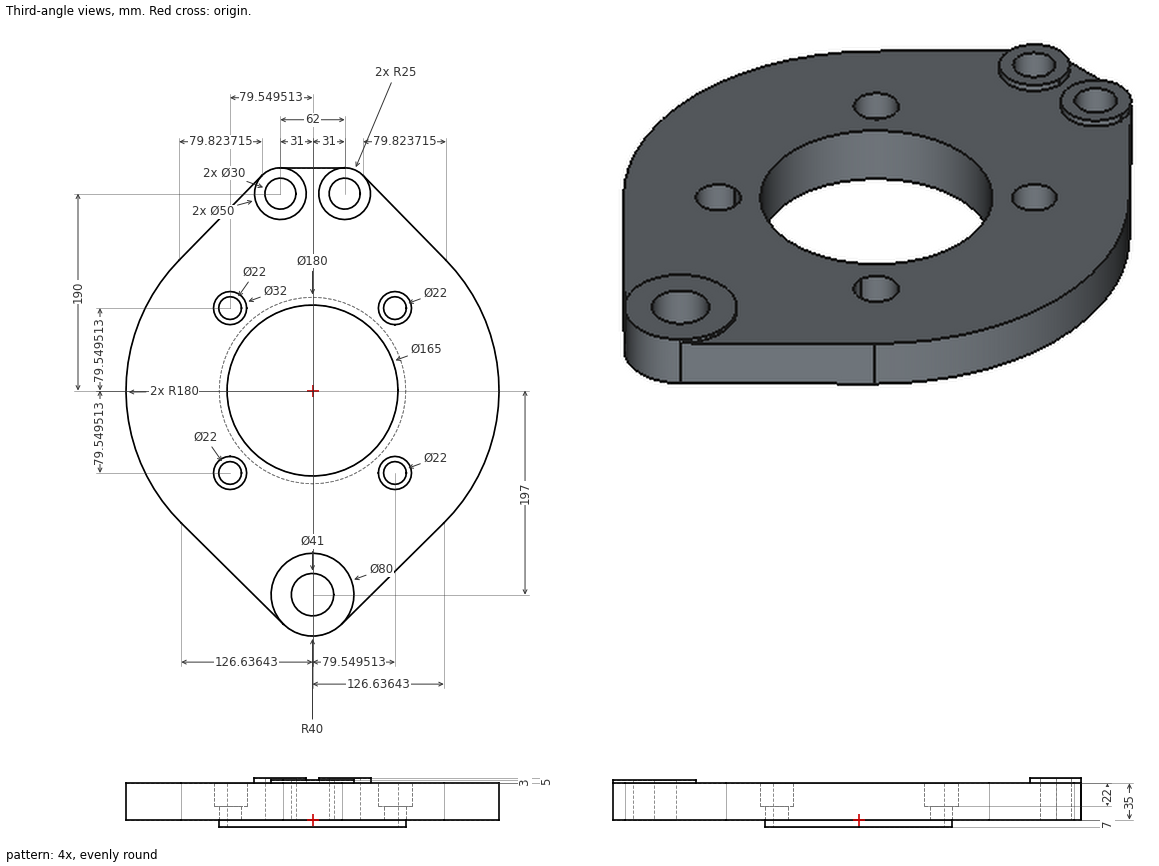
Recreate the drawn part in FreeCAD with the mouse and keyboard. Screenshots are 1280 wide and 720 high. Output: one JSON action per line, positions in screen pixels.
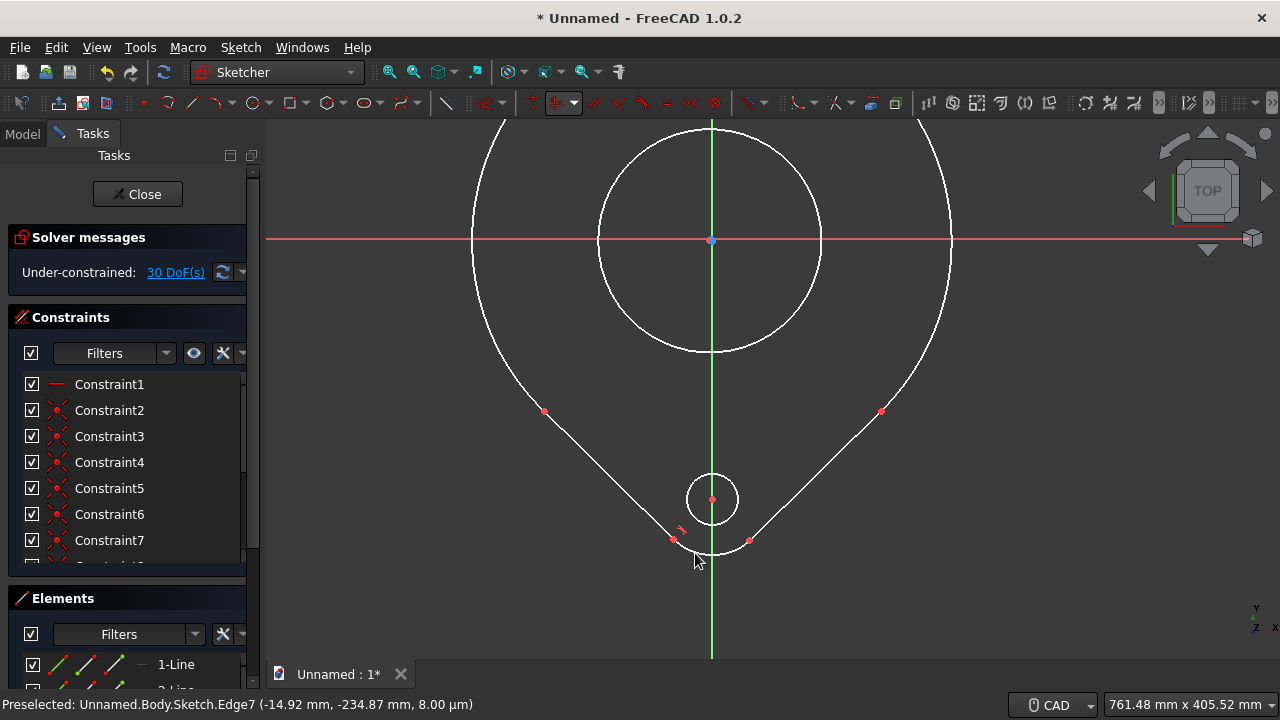
{"action": "left_click", "coordinate": [789, 502]}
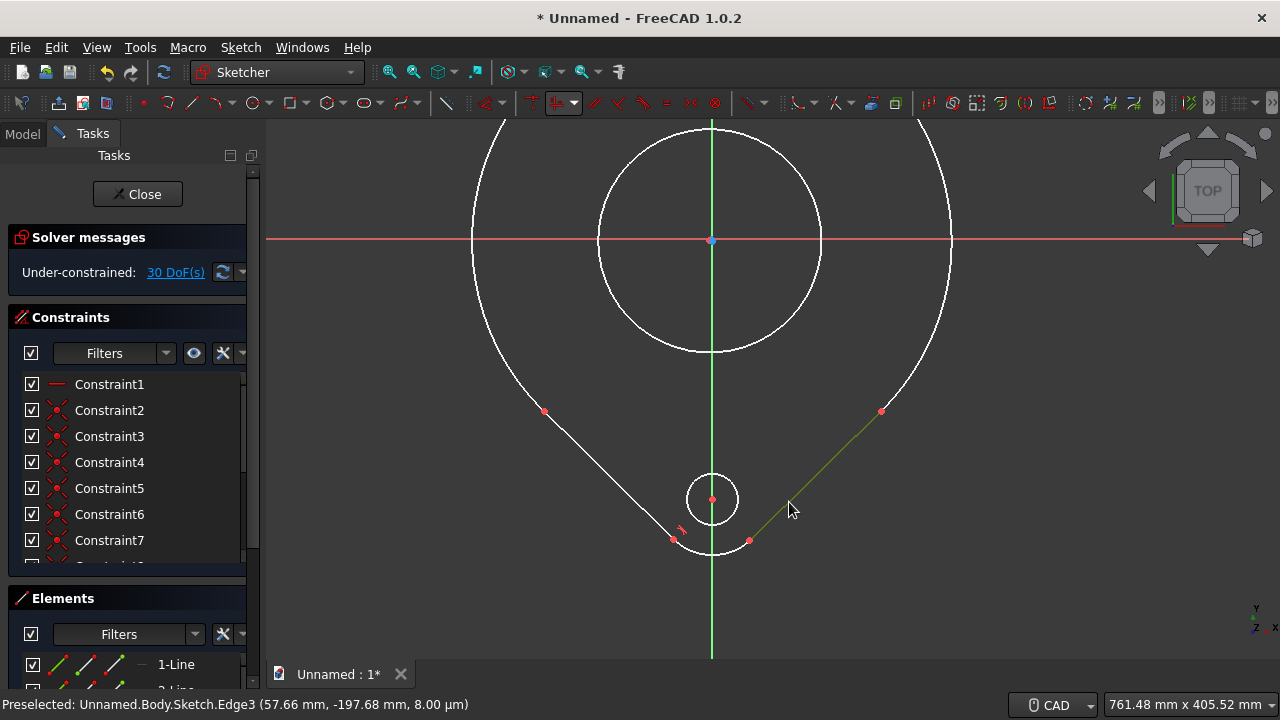
{"action": "left_click", "coordinate": [695, 552]}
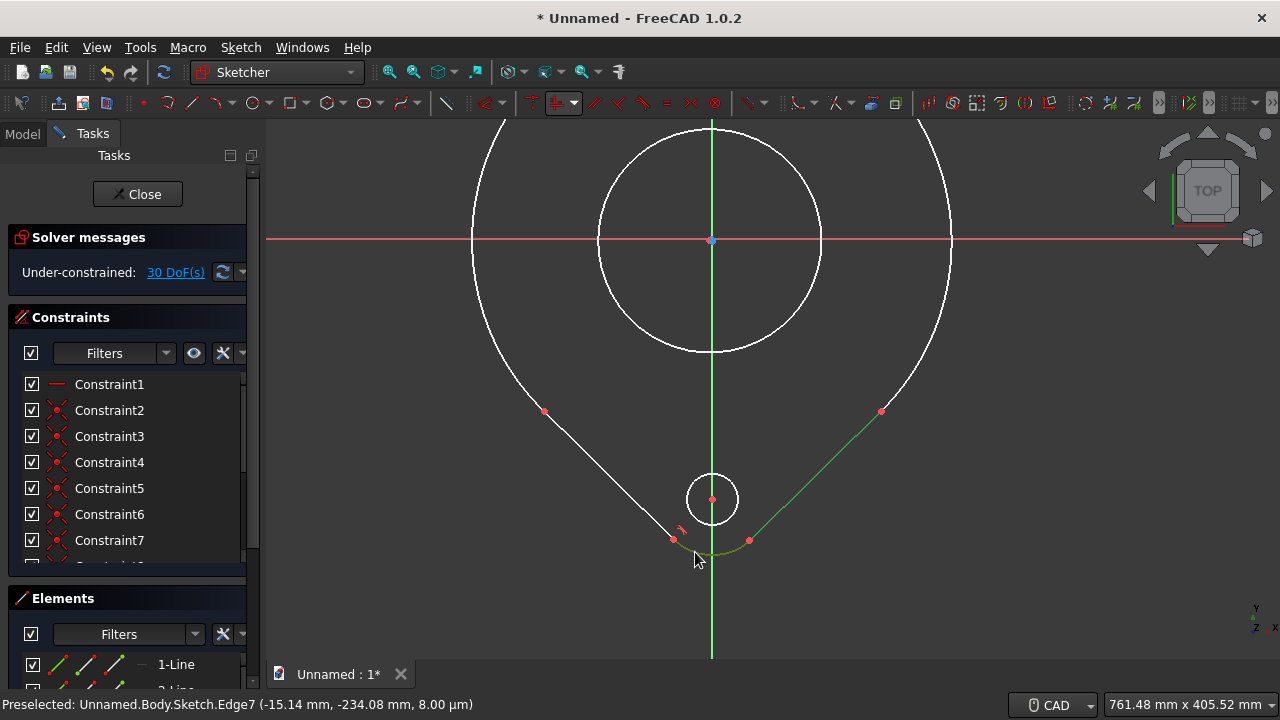
{"action": "key", "text": "t"}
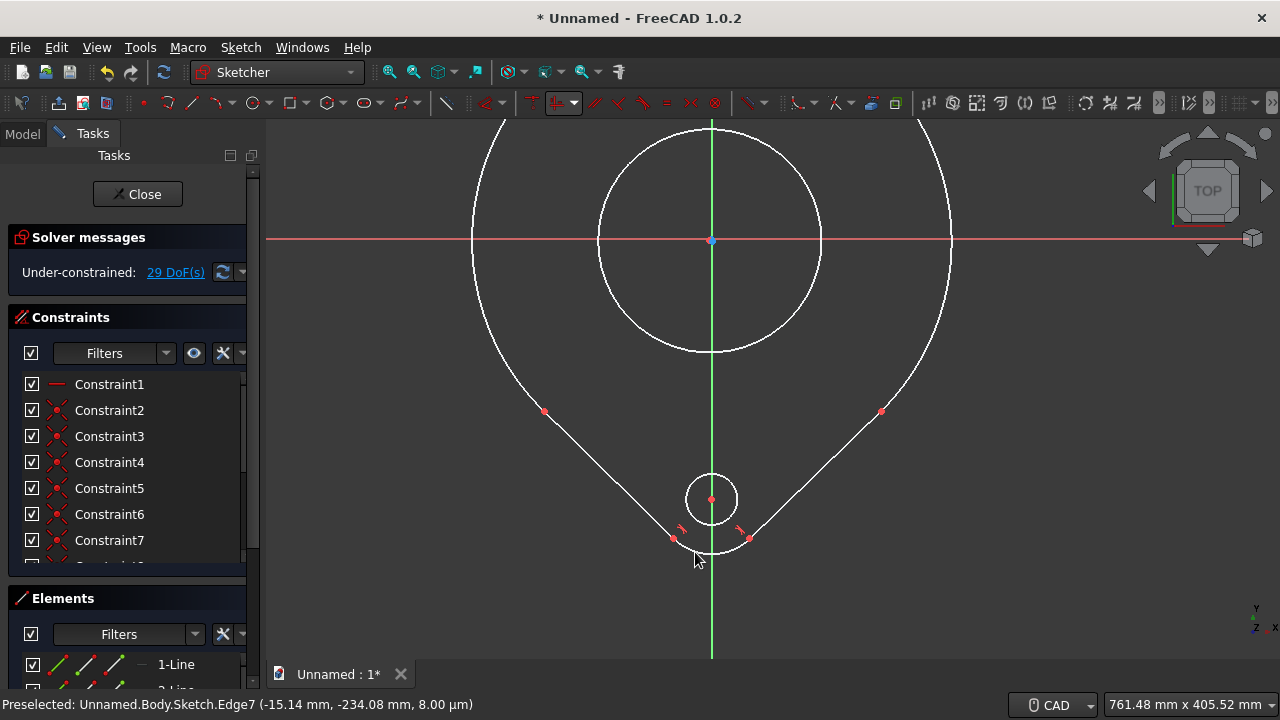
{"action": "scroll", "coordinate": [696, 553], "scroll_direction": "down", "scroll_amount": 3}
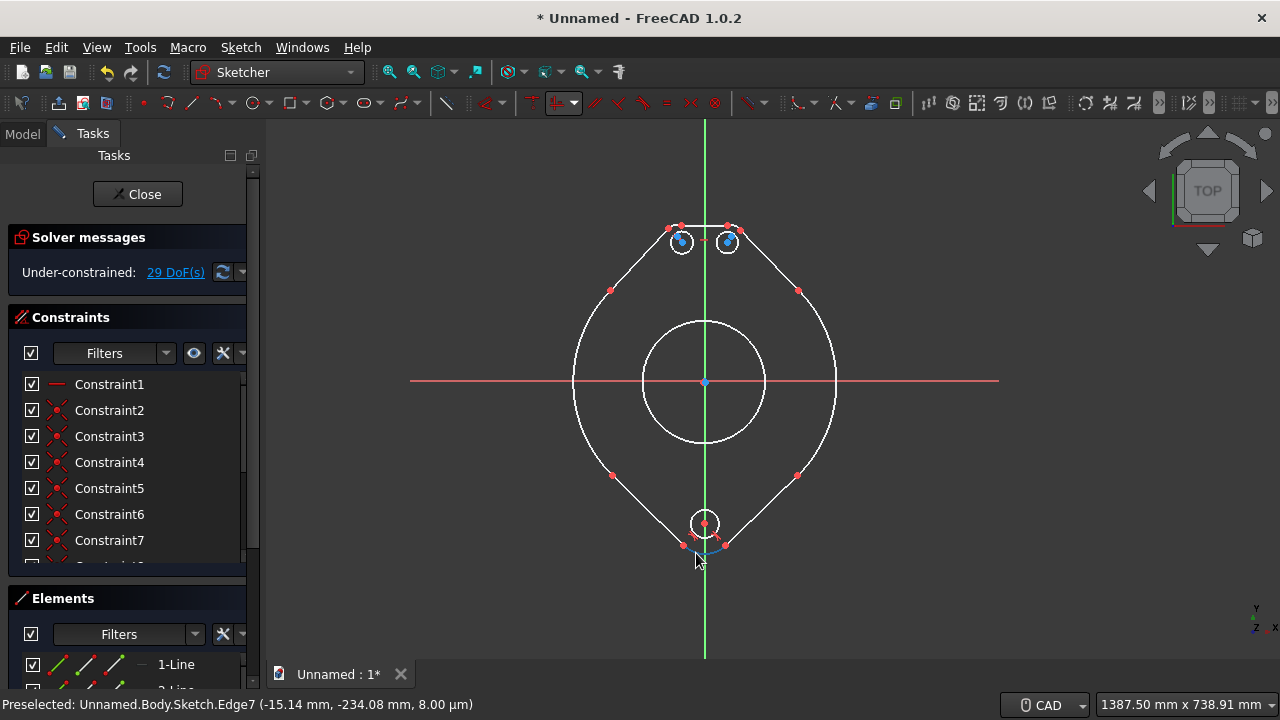
{"action": "left_click", "coordinate": [781, 273]}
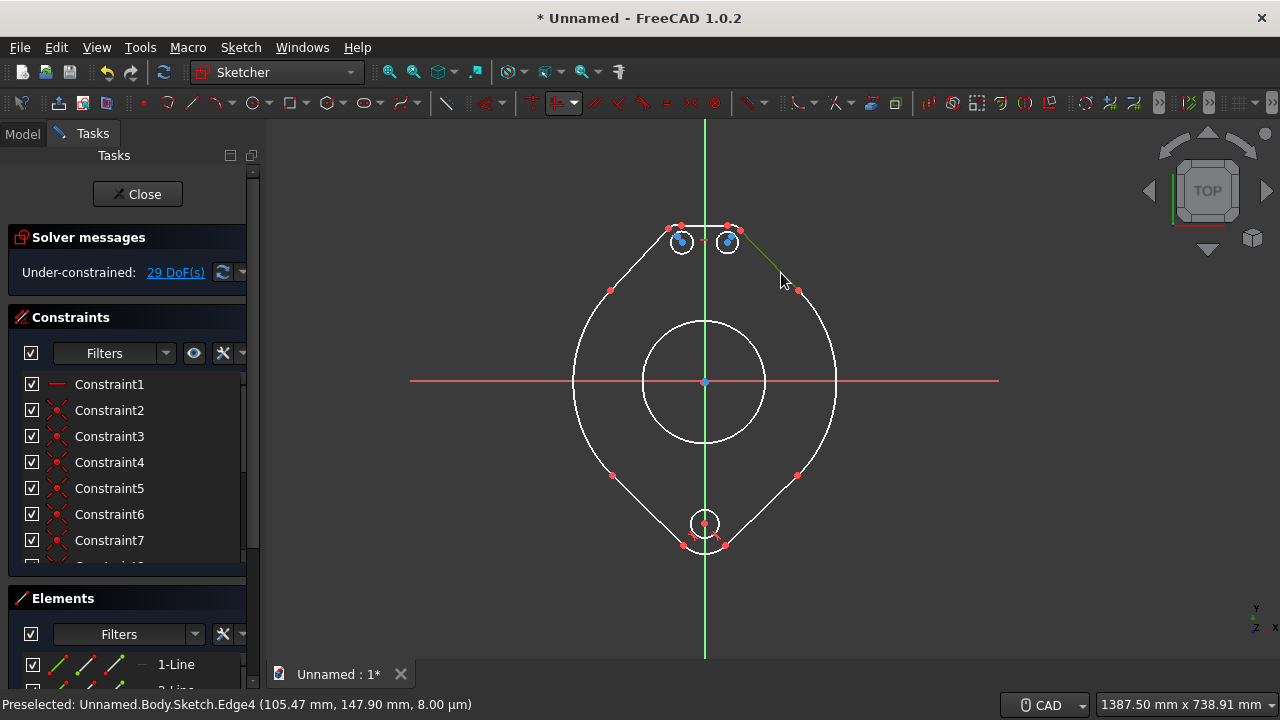
{"action": "scroll", "coordinate": [735, 226], "scroll_direction": "up", "scroll_amount": 4}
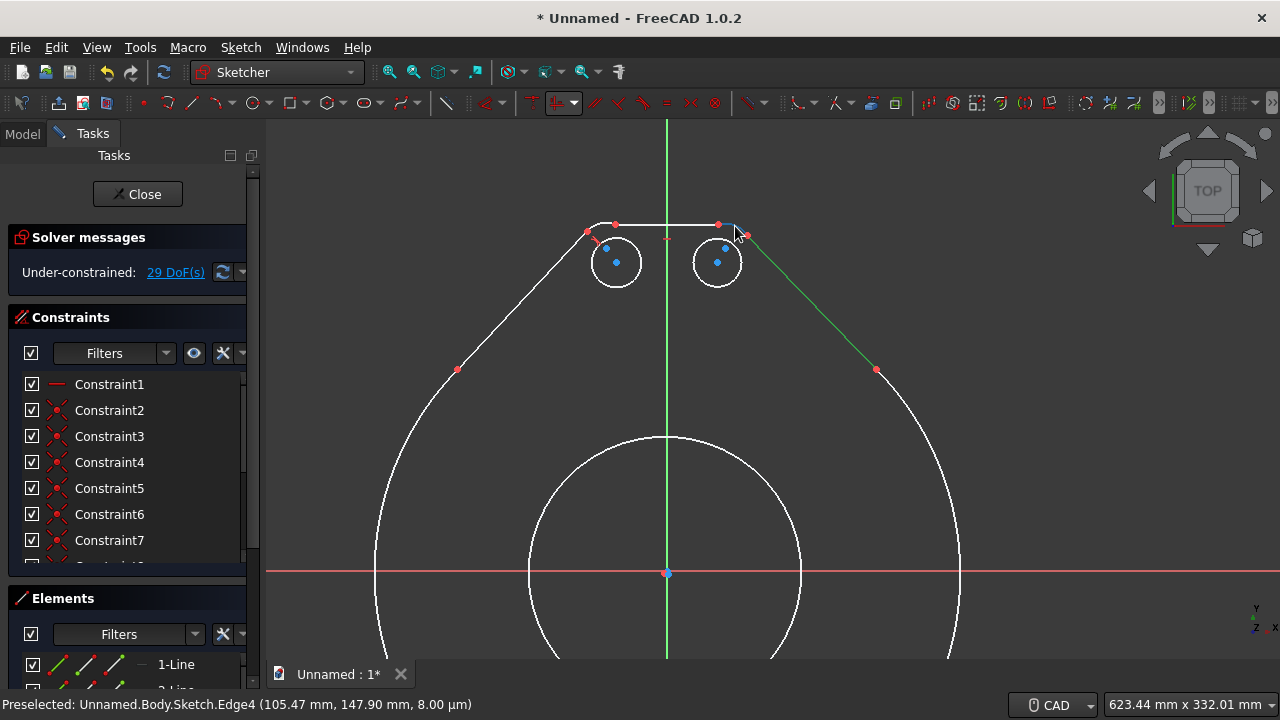
{"action": "left_click", "coordinate": [735, 225]}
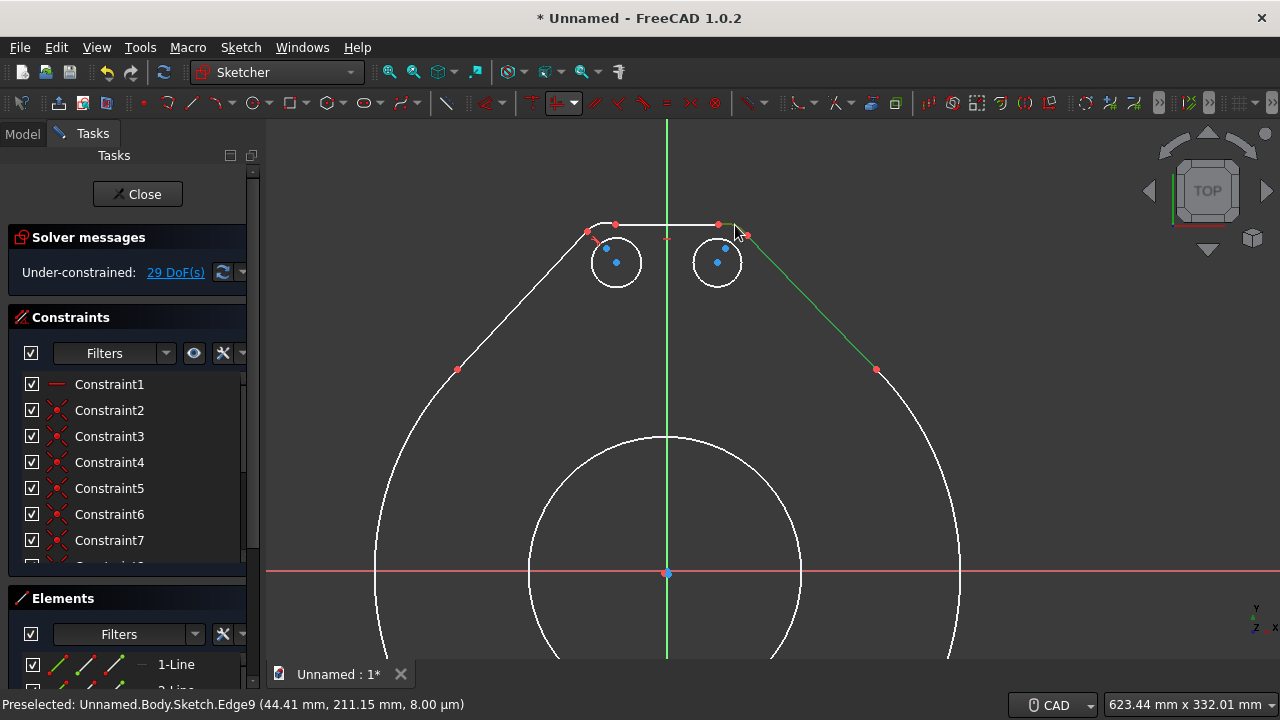
{"action": "left_click", "coordinate": [644, 104]}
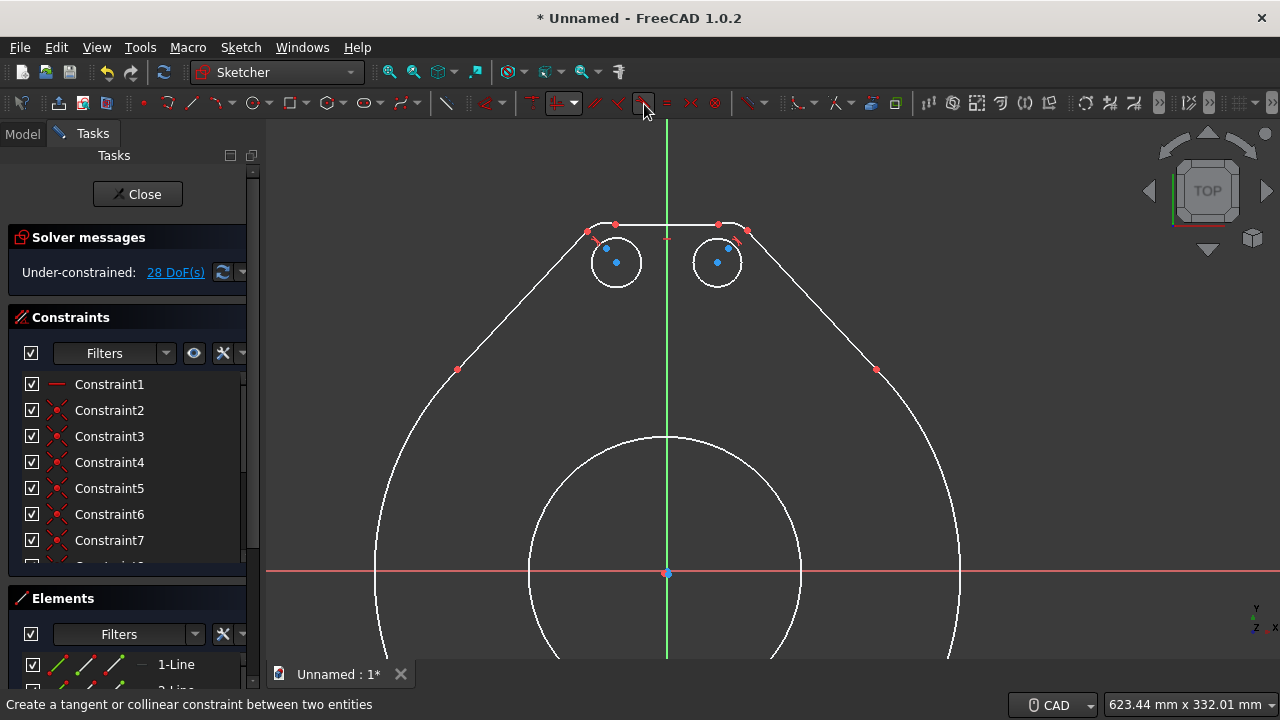
{"action": "left_click", "coordinate": [688, 225]}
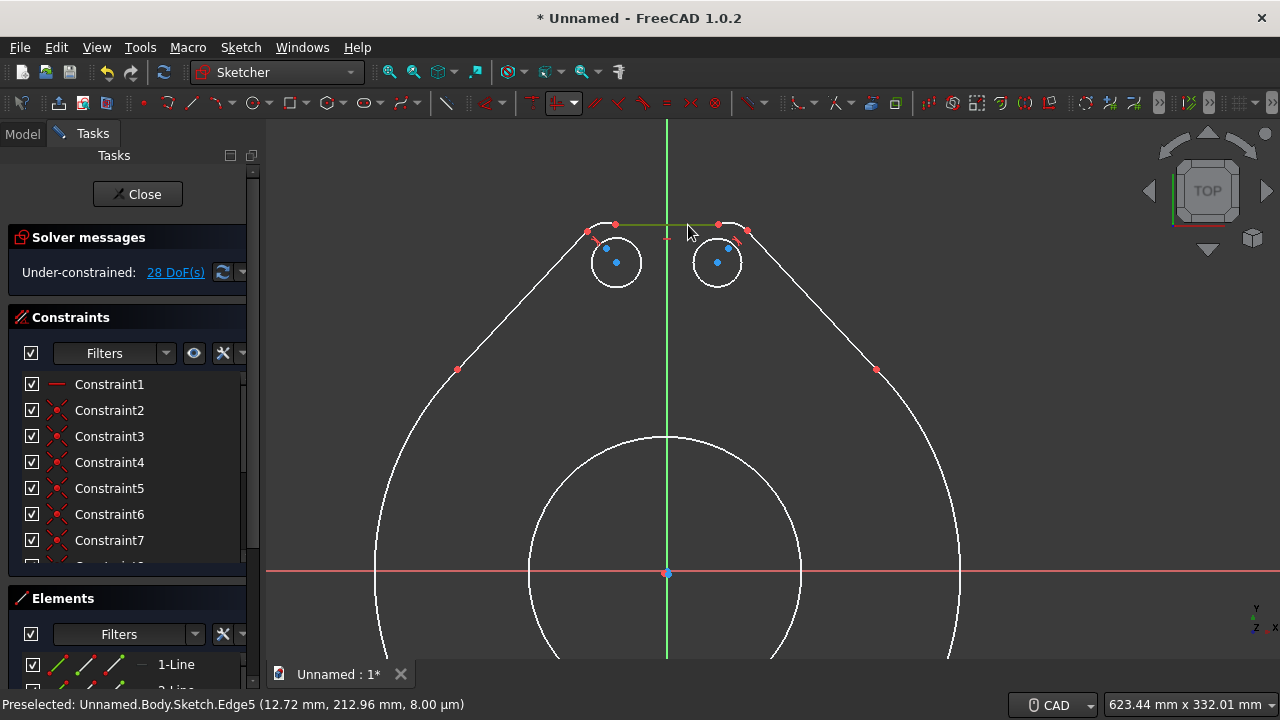
{"action": "scroll", "coordinate": [740, 225], "scroll_direction": "up", "scroll_amount": 2}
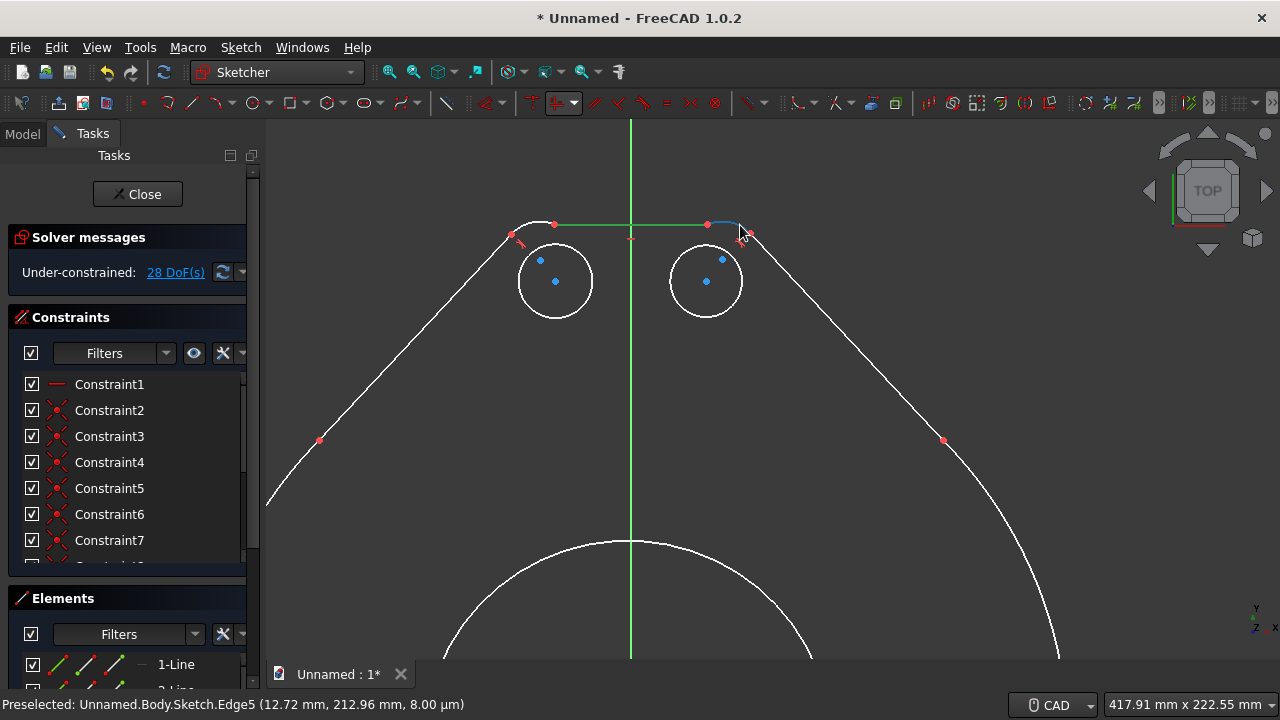
{"action": "left_click", "coordinate": [739, 225]}